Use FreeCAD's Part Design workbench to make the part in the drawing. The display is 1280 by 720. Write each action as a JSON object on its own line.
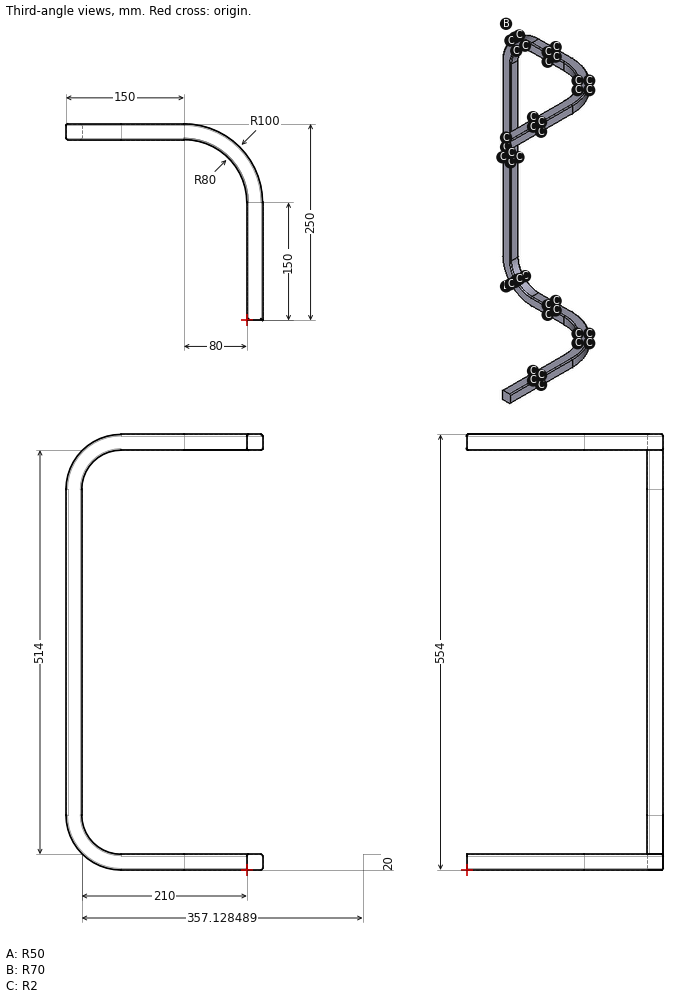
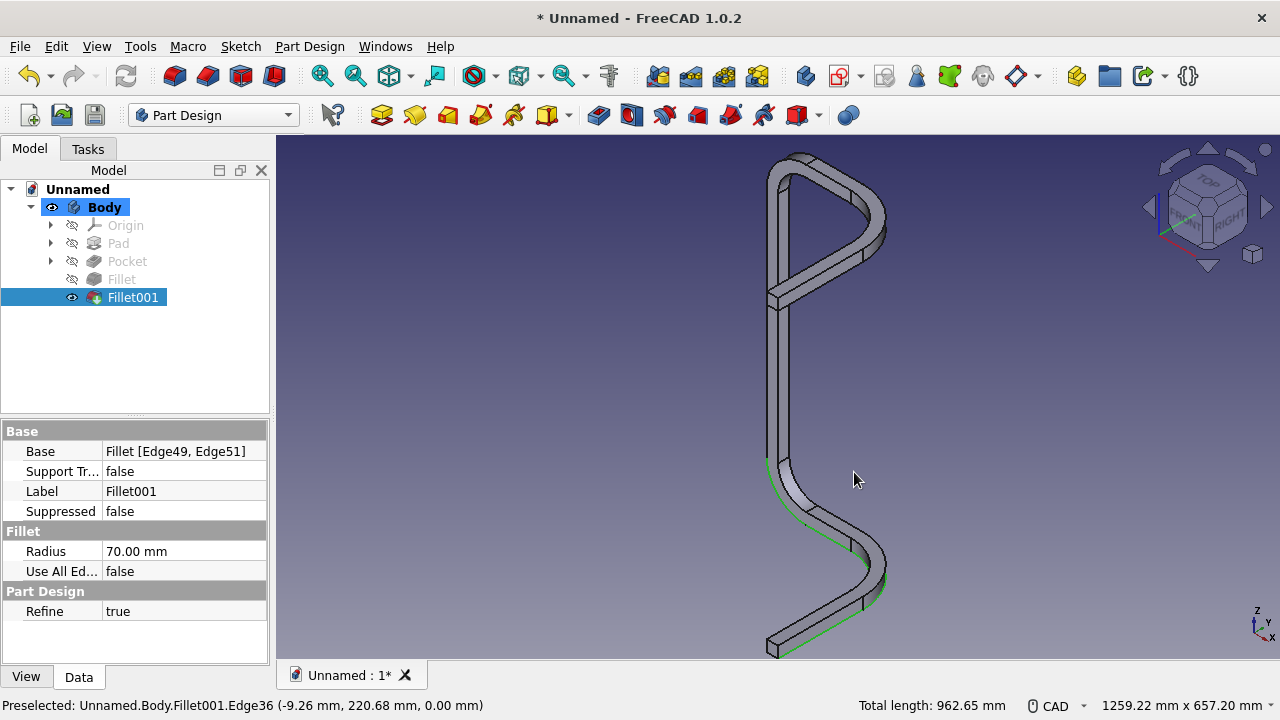
{"action": "left_click", "coordinate": [323, 76]}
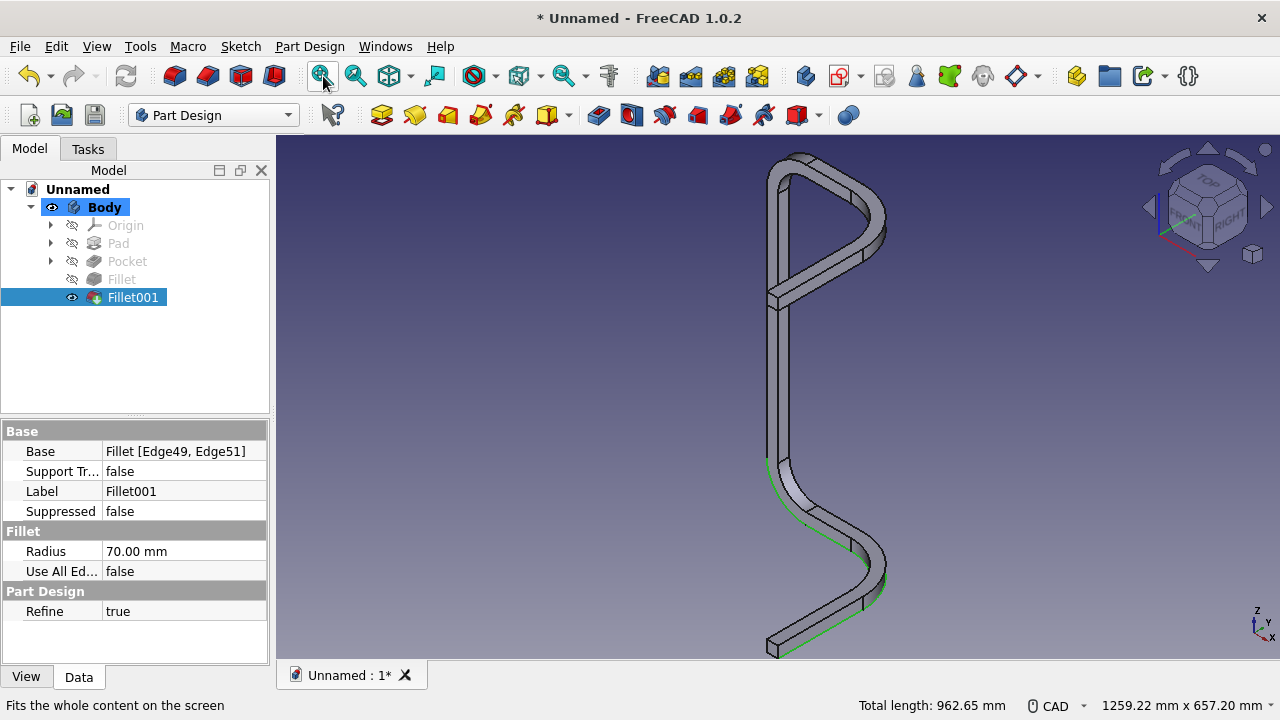
{"action": "left_click", "coordinate": [886, 216], "text": "ctrl"}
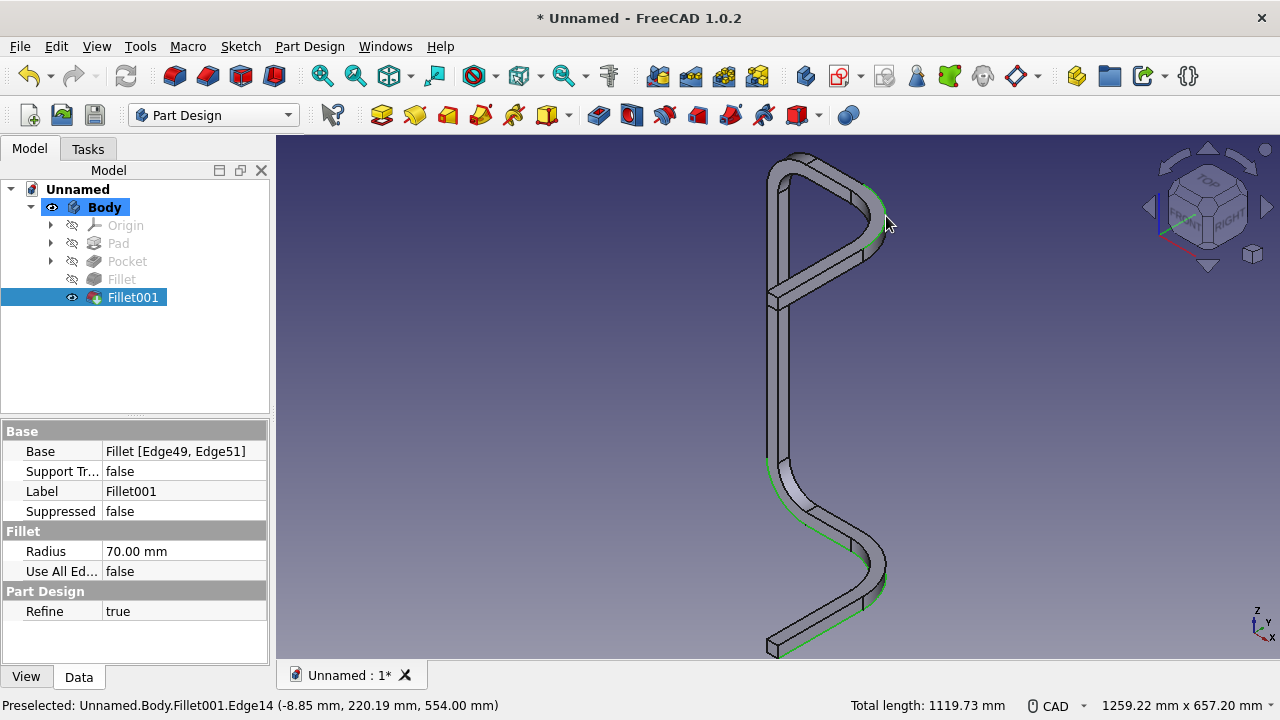
{"action": "left_click", "coordinate": [870, 216], "text": "ctrl"}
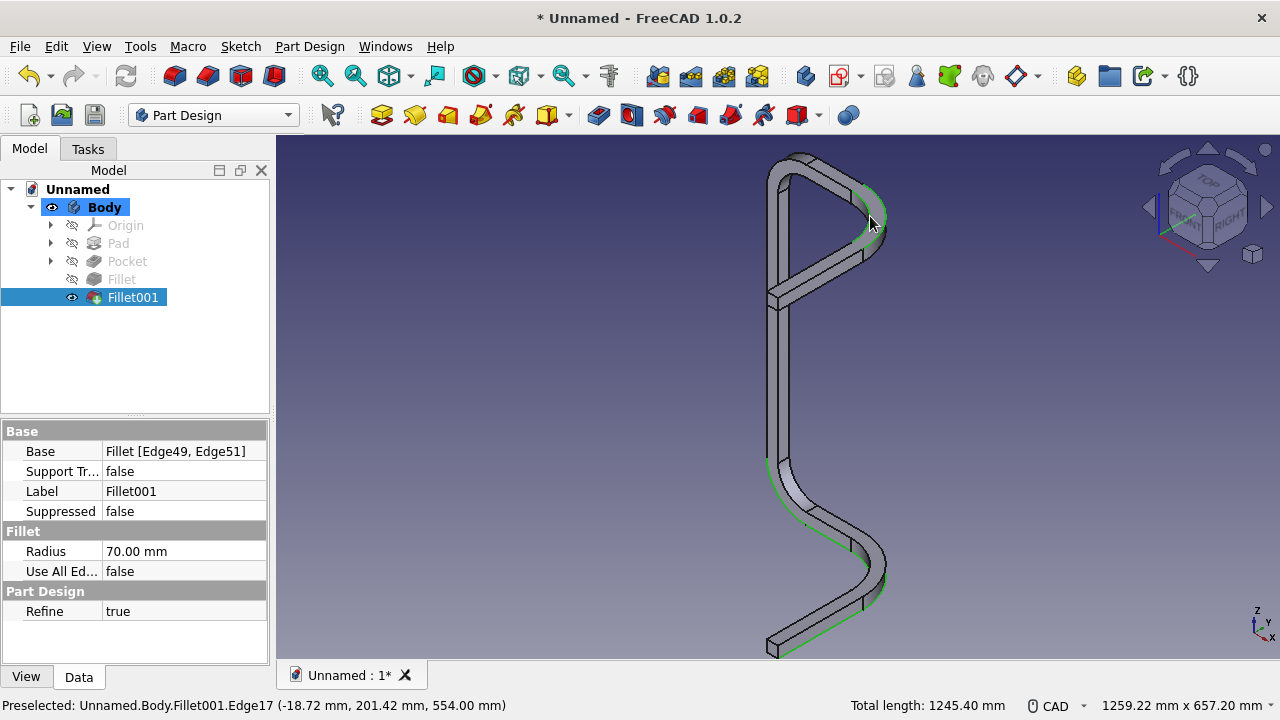
{"action": "left_click", "coordinate": [886, 563], "text": "ctrl"}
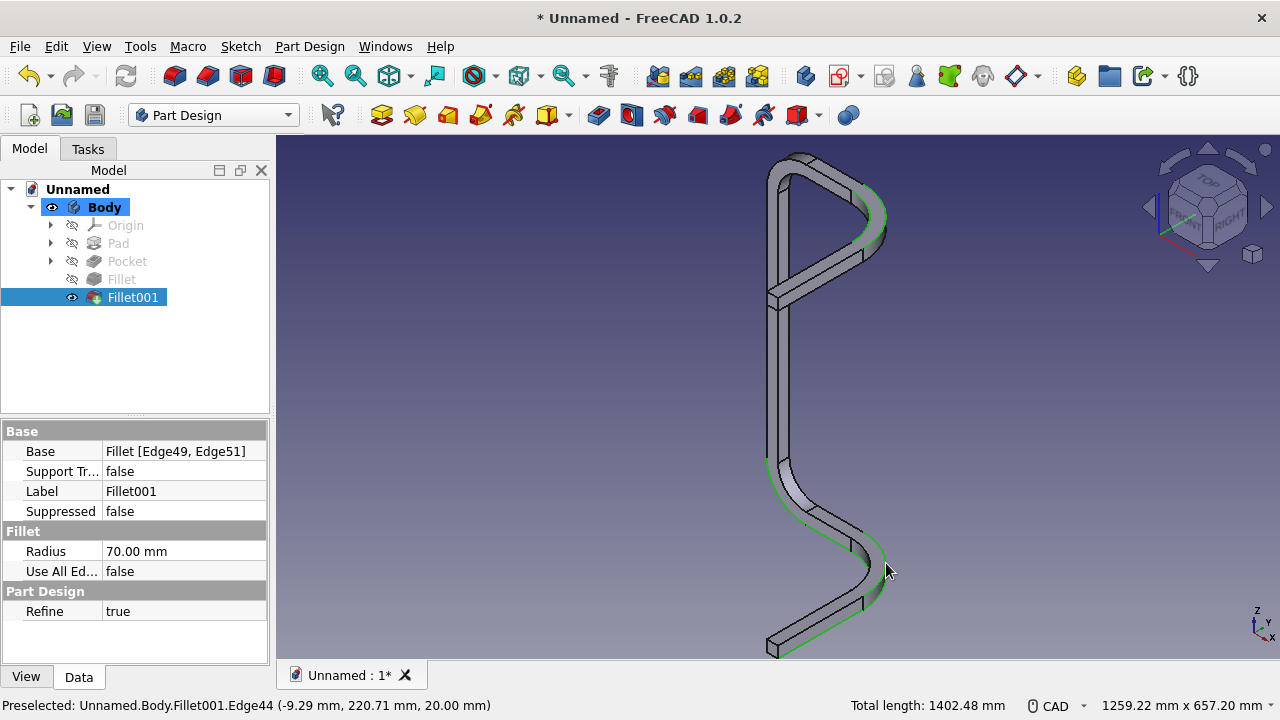
{"action": "left_click", "coordinate": [820, 620], "text": "ctrl"}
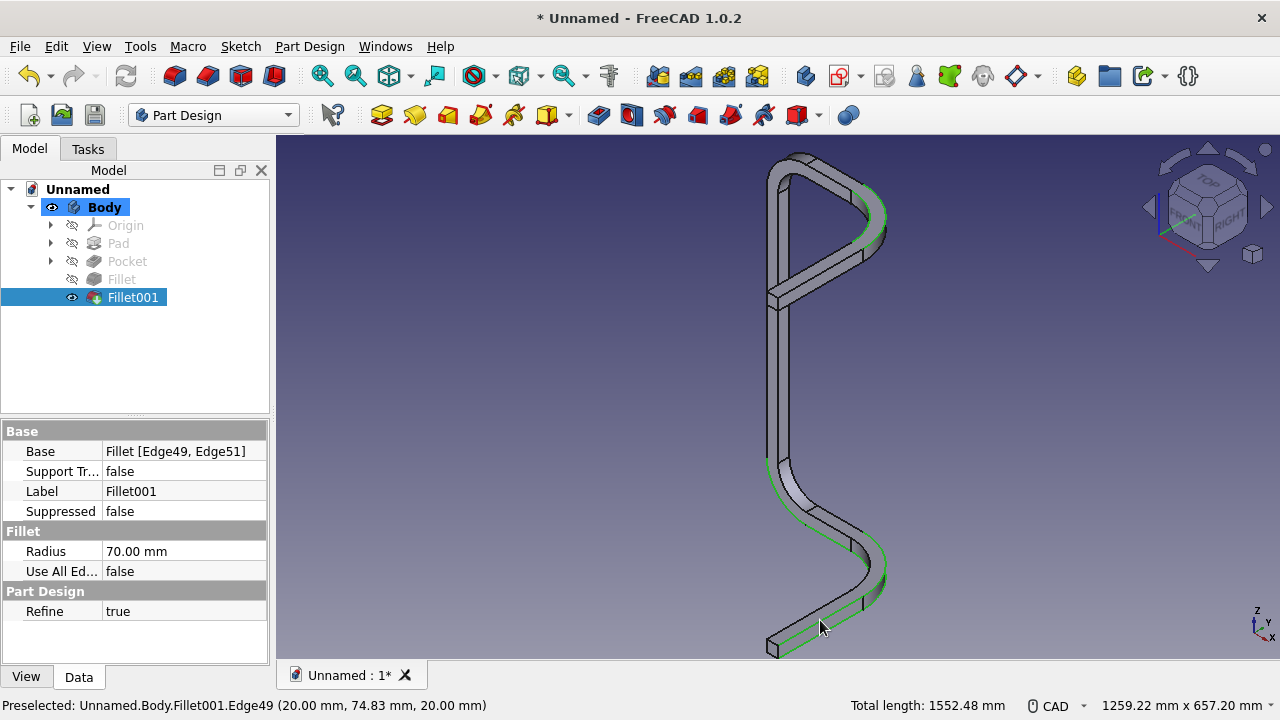
{"action": "left_click", "coordinate": [869, 558], "text": "ctrl"}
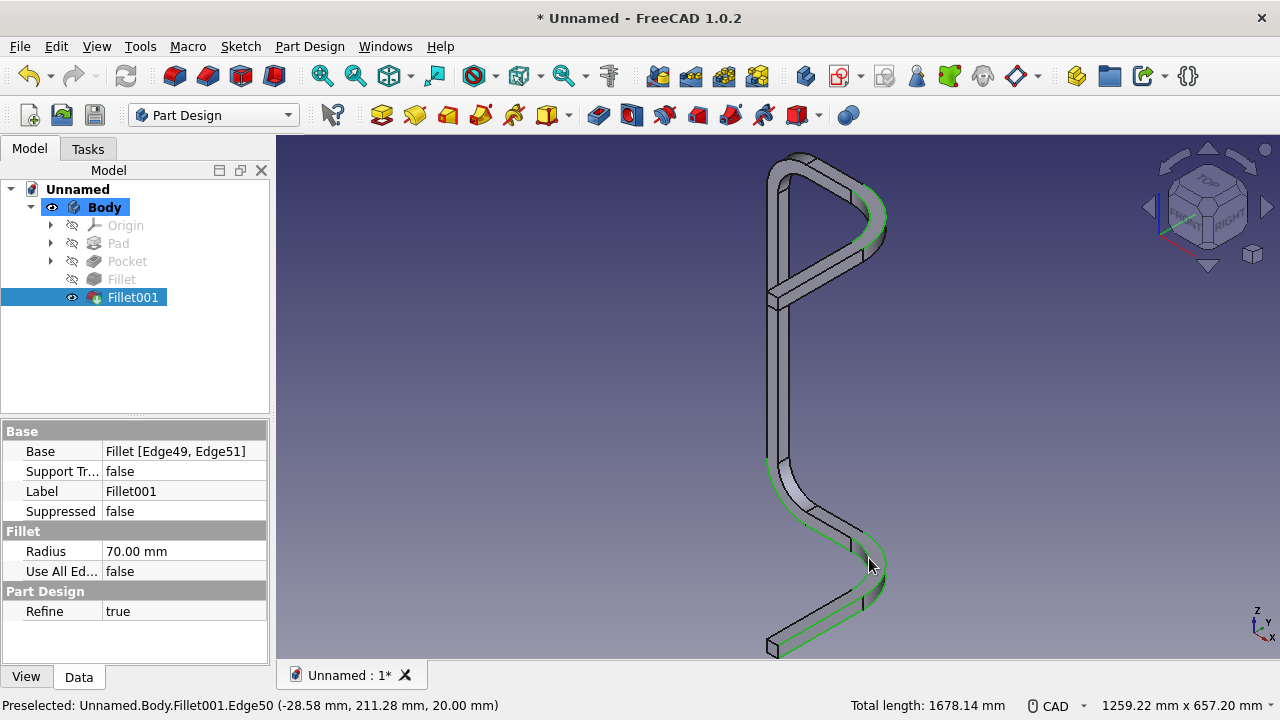
{"action": "left_click", "coordinate": [829, 524], "text": "ctrl"}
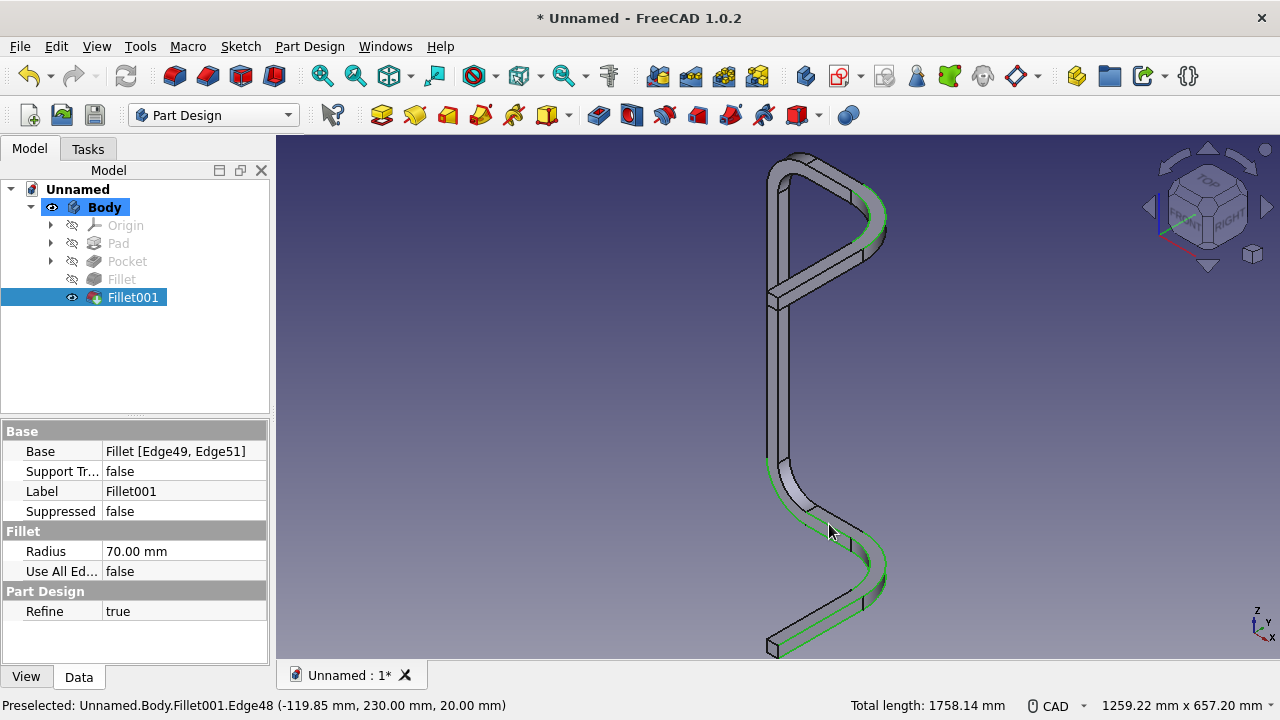
{"action": "left_click", "coordinate": [772, 294], "text": "ctrl"}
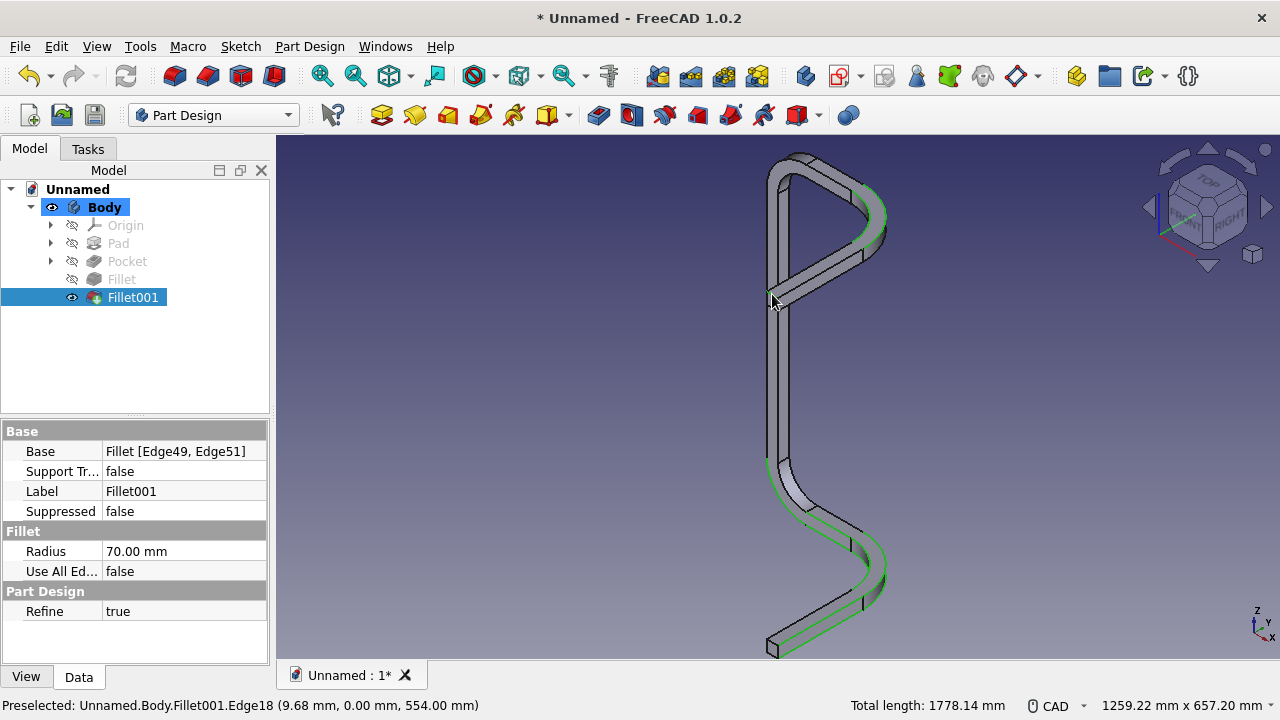
{"action": "left_click", "coordinate": [778, 328], "text": "ctrl"}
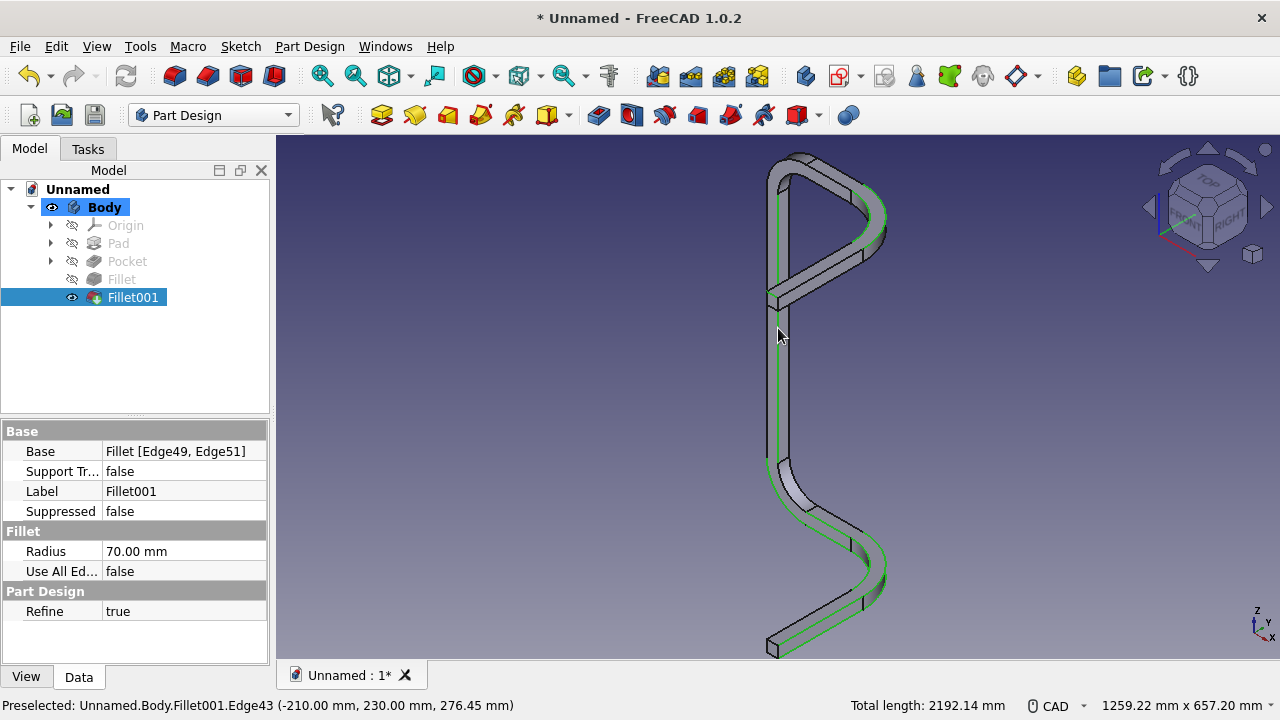
{"action": "left_click", "coordinate": [809, 498], "text": "ctrl"}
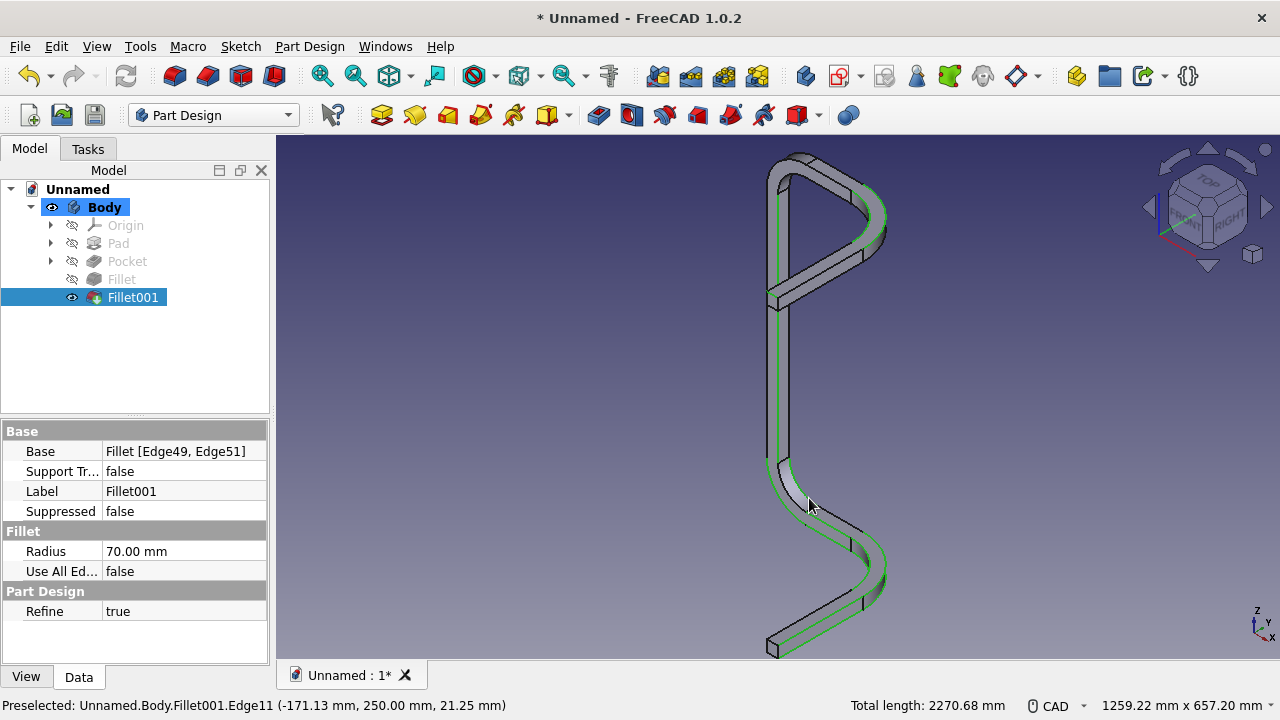
{"action": "left_click", "coordinate": [786, 490], "text": "ctrl"}